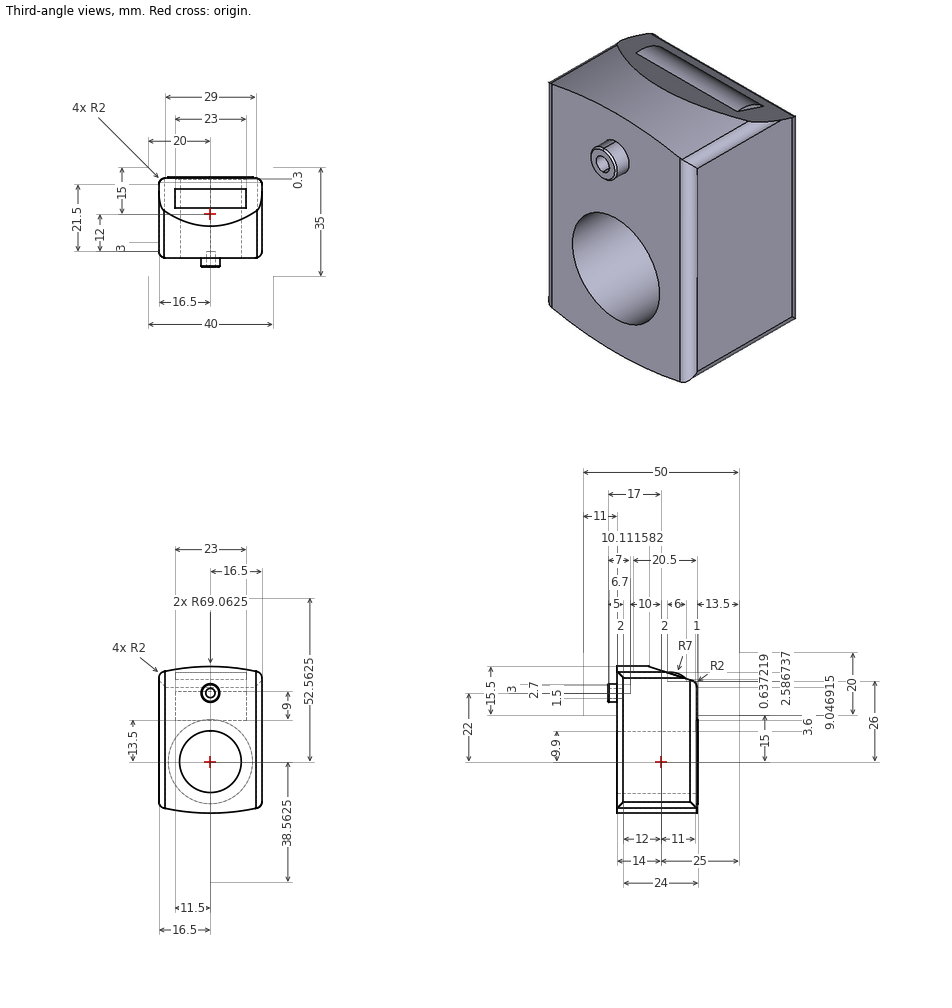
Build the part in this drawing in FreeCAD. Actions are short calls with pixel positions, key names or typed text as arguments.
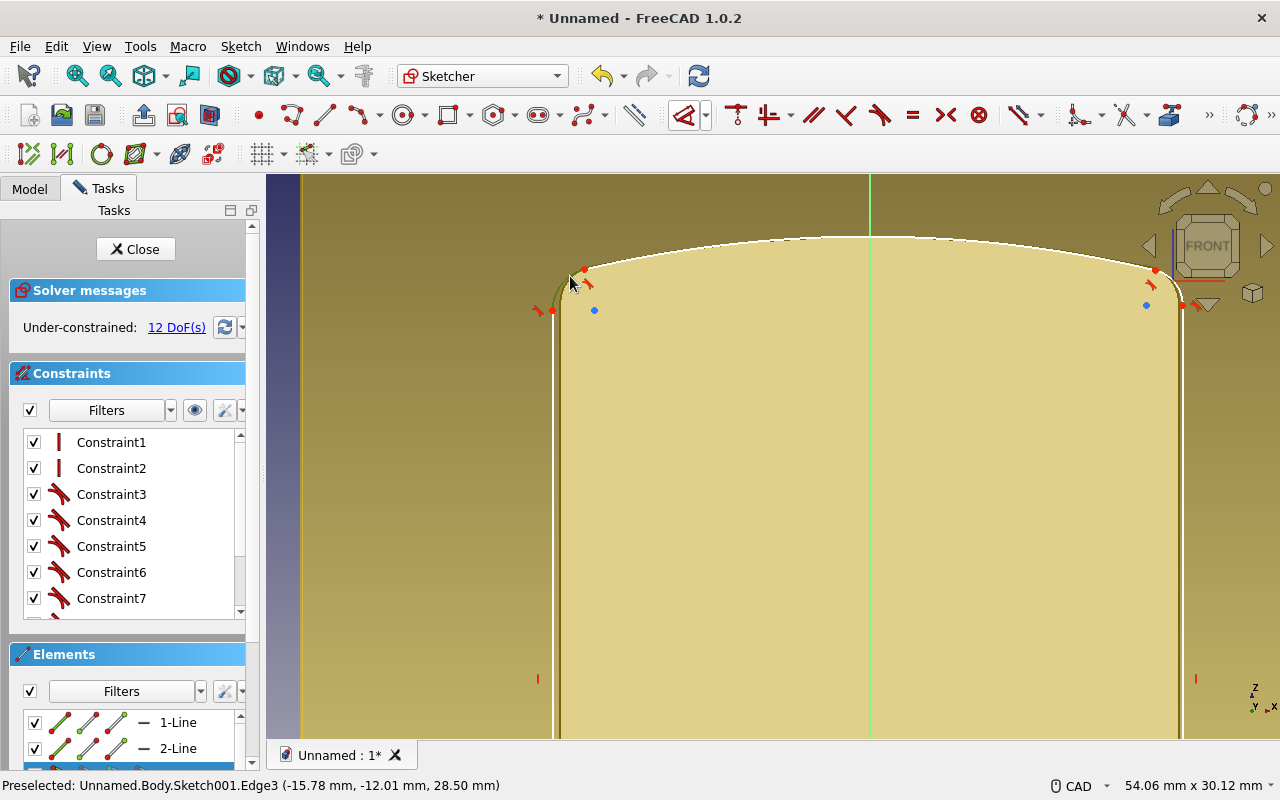
scroll(570, 276, down, 4)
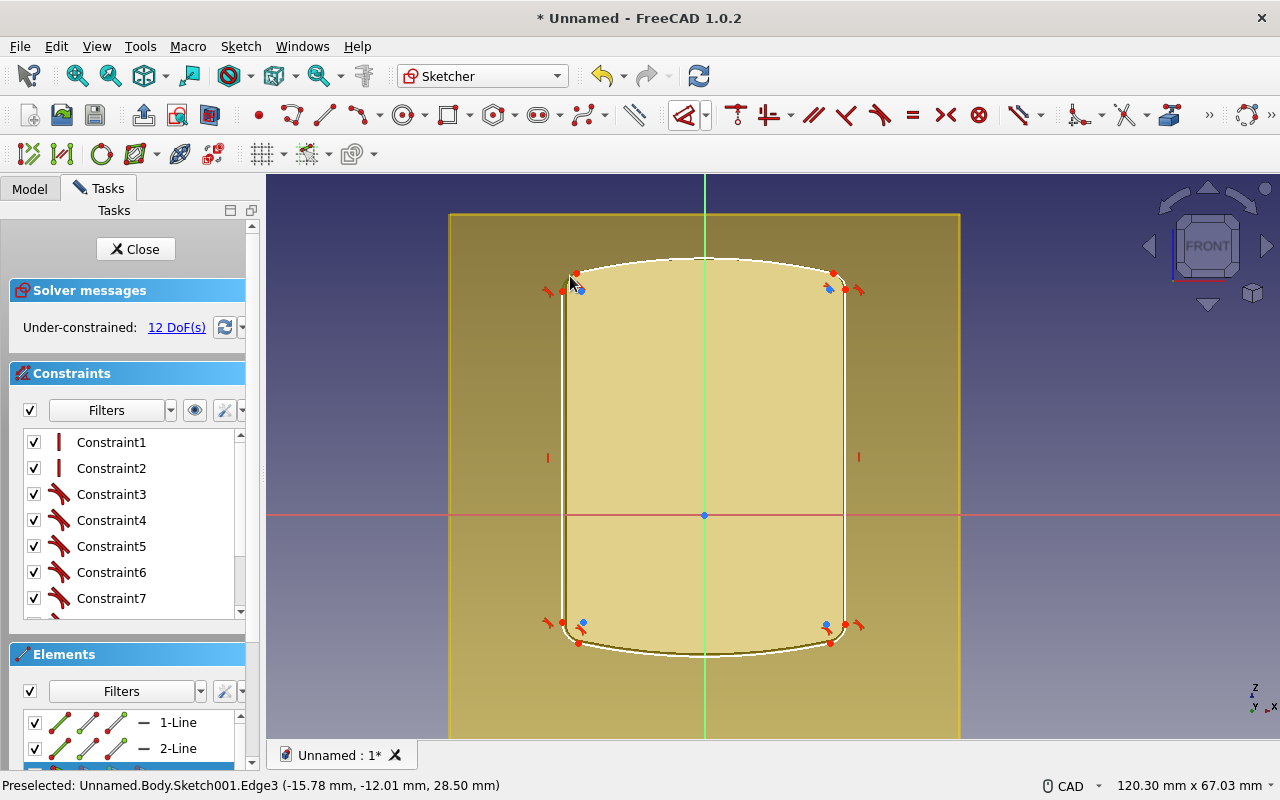
scroll(844, 283, up, 4)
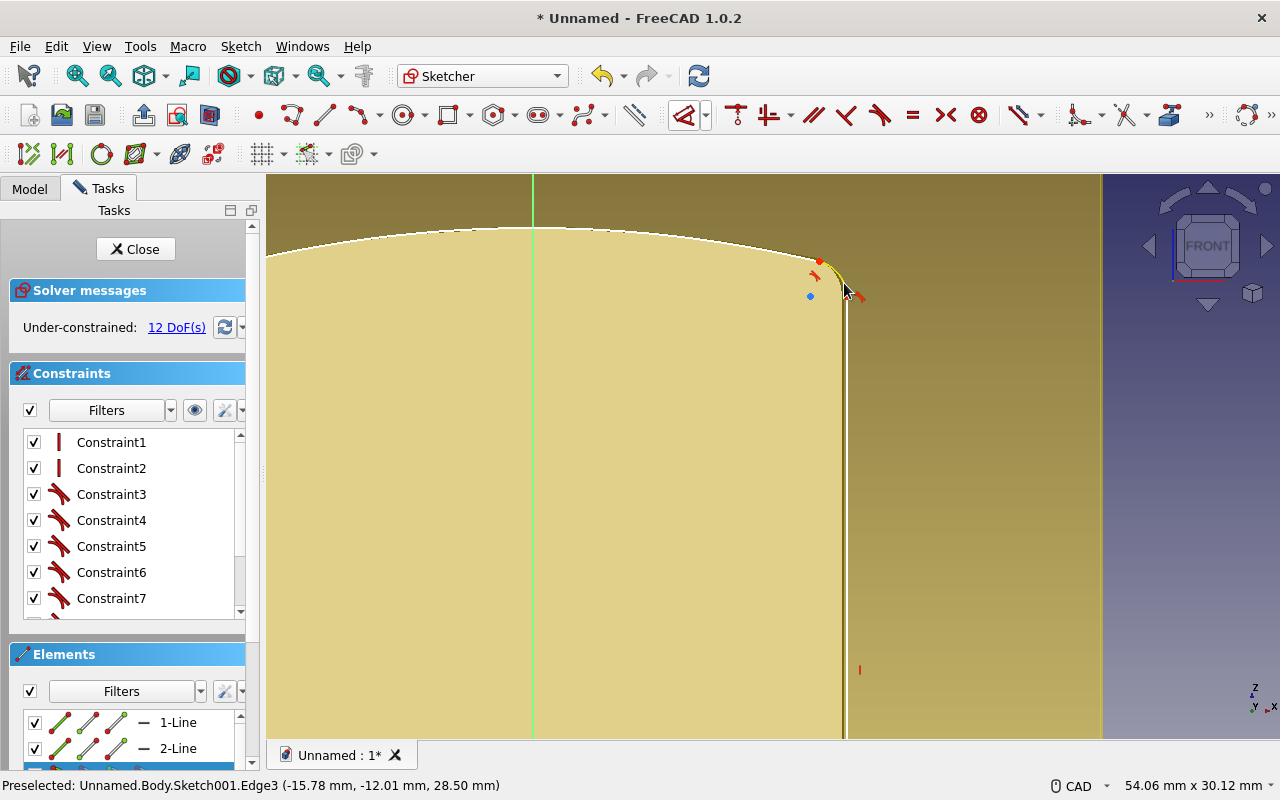
click(844, 283)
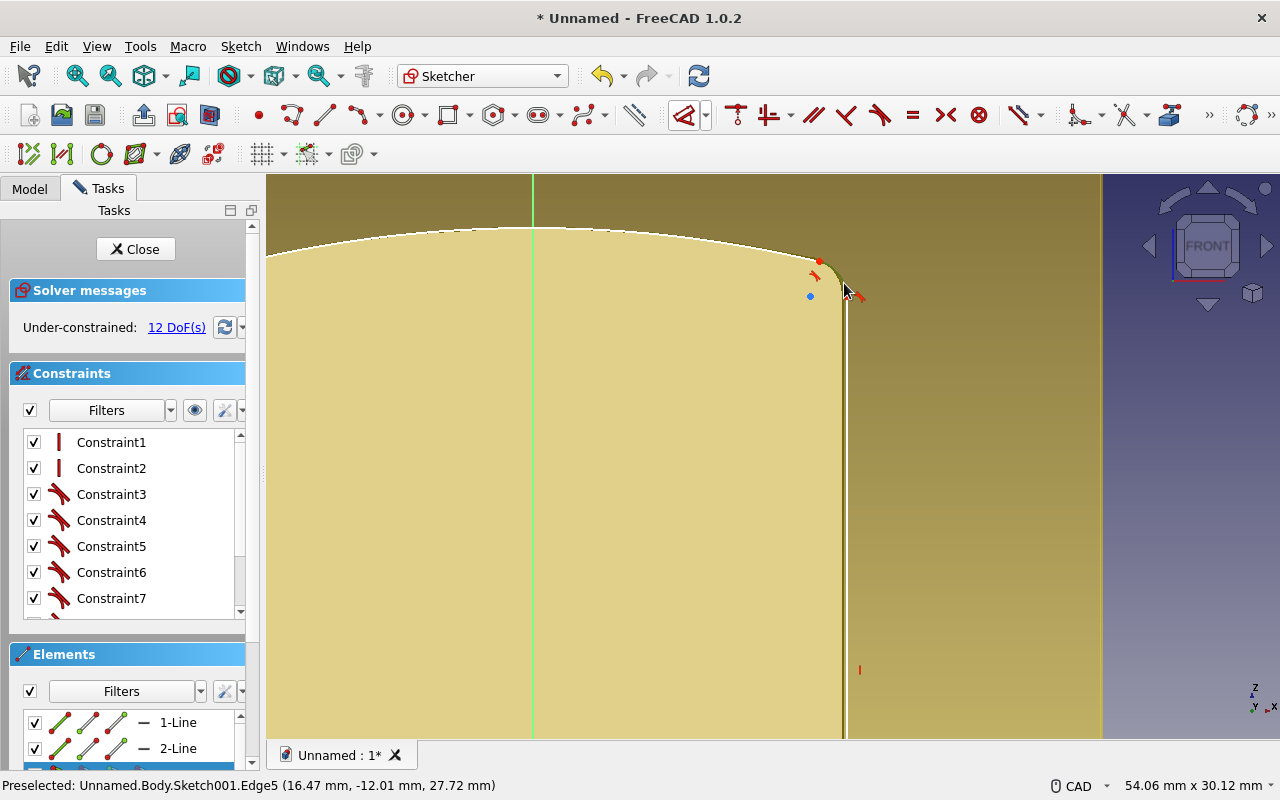
scroll(844, 283, down, 4)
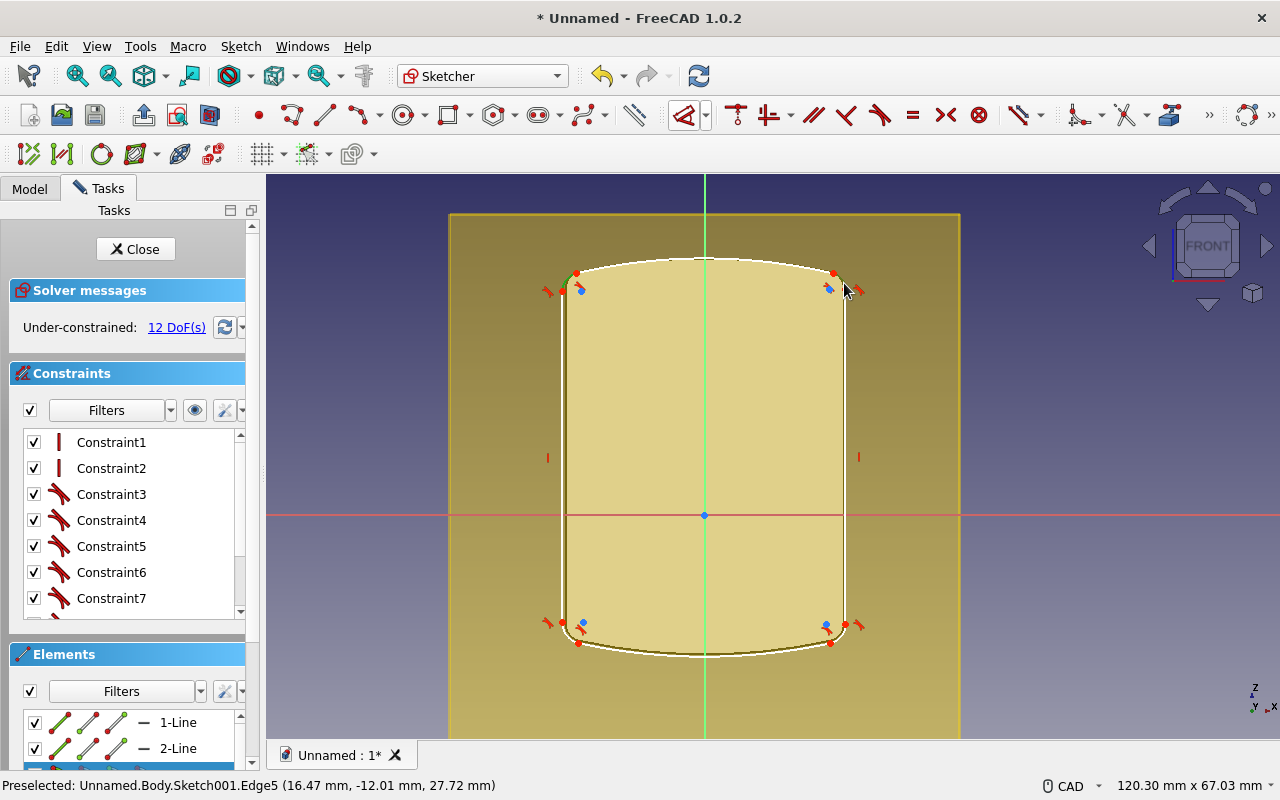
scroll(837, 640, up, 3)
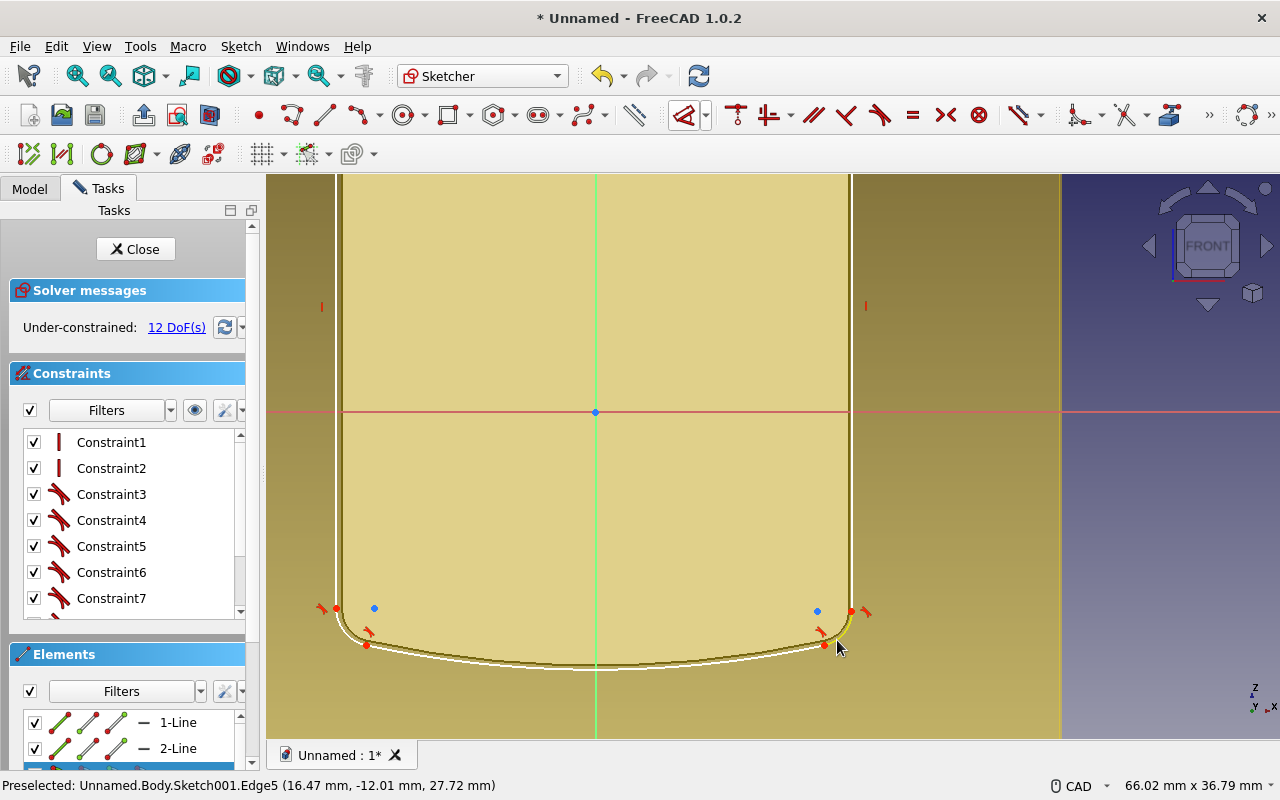
click(837, 640)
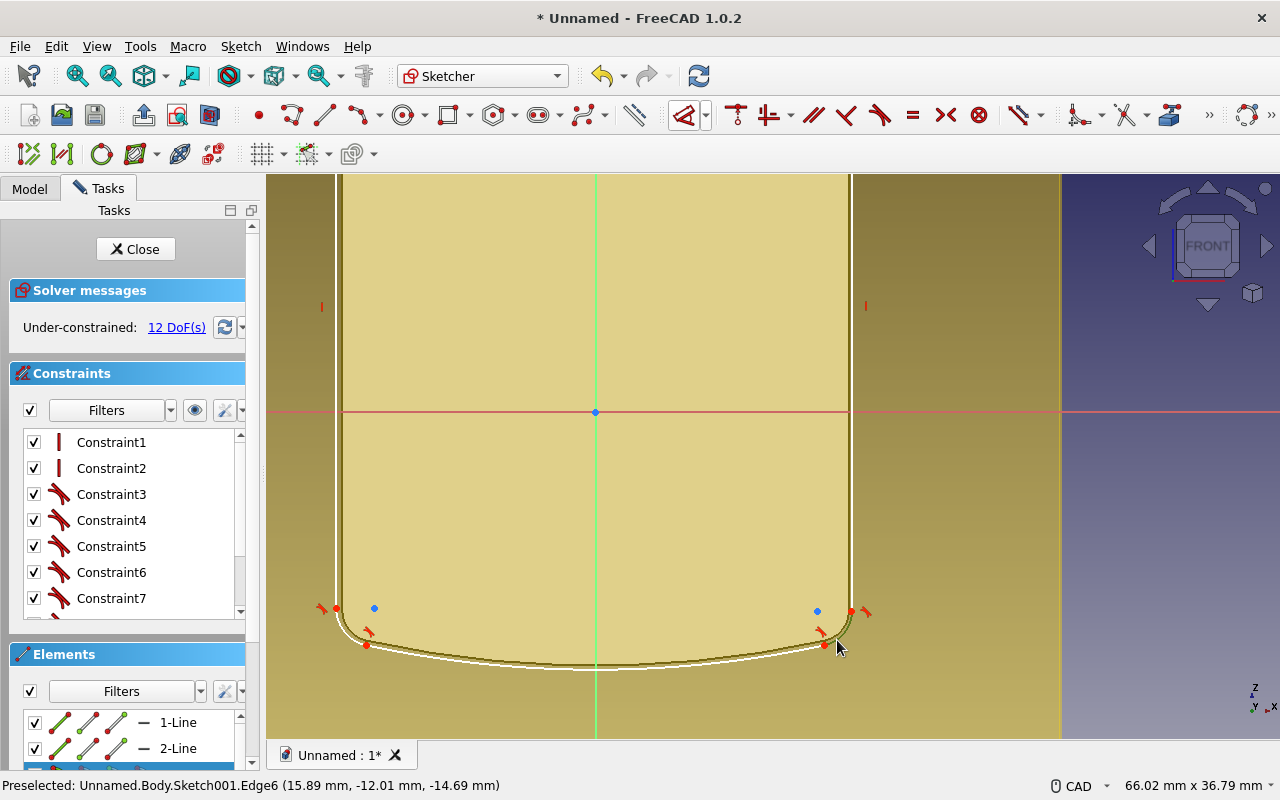
click(339, 623)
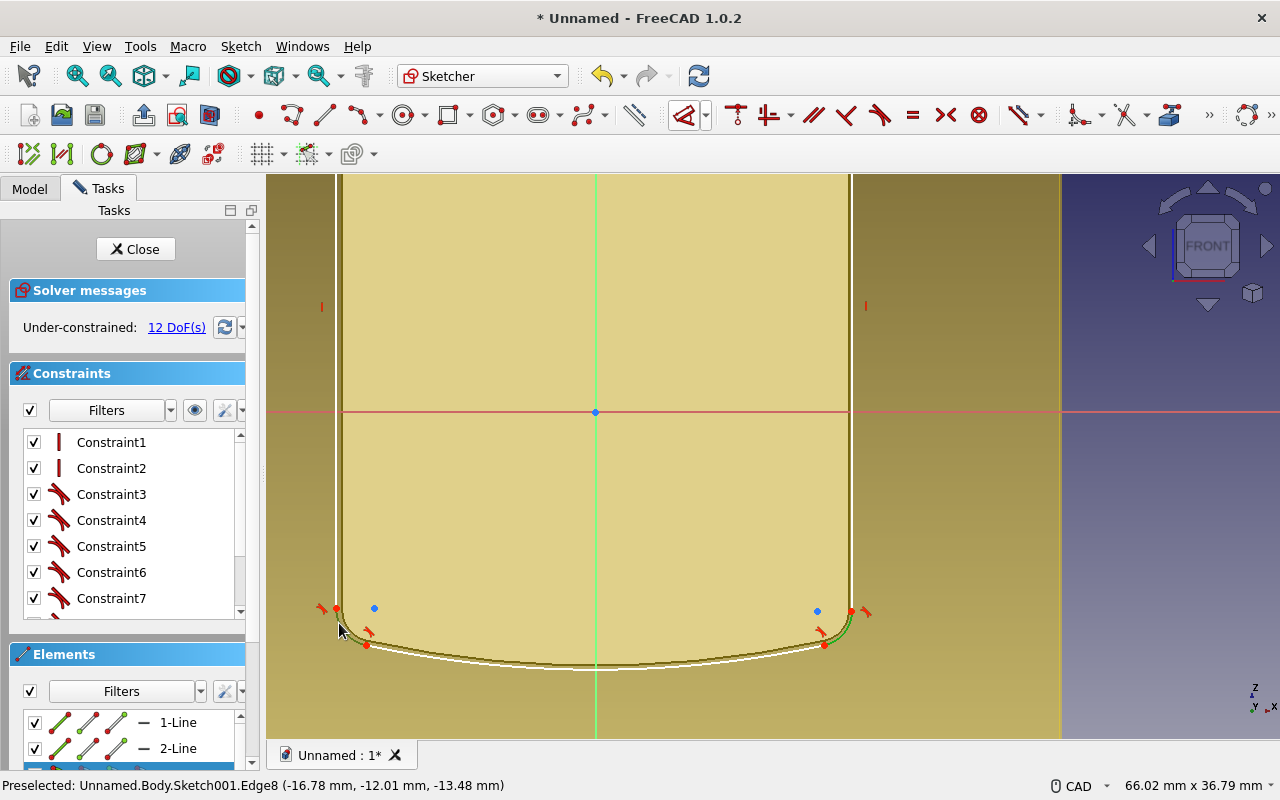
click(913, 116)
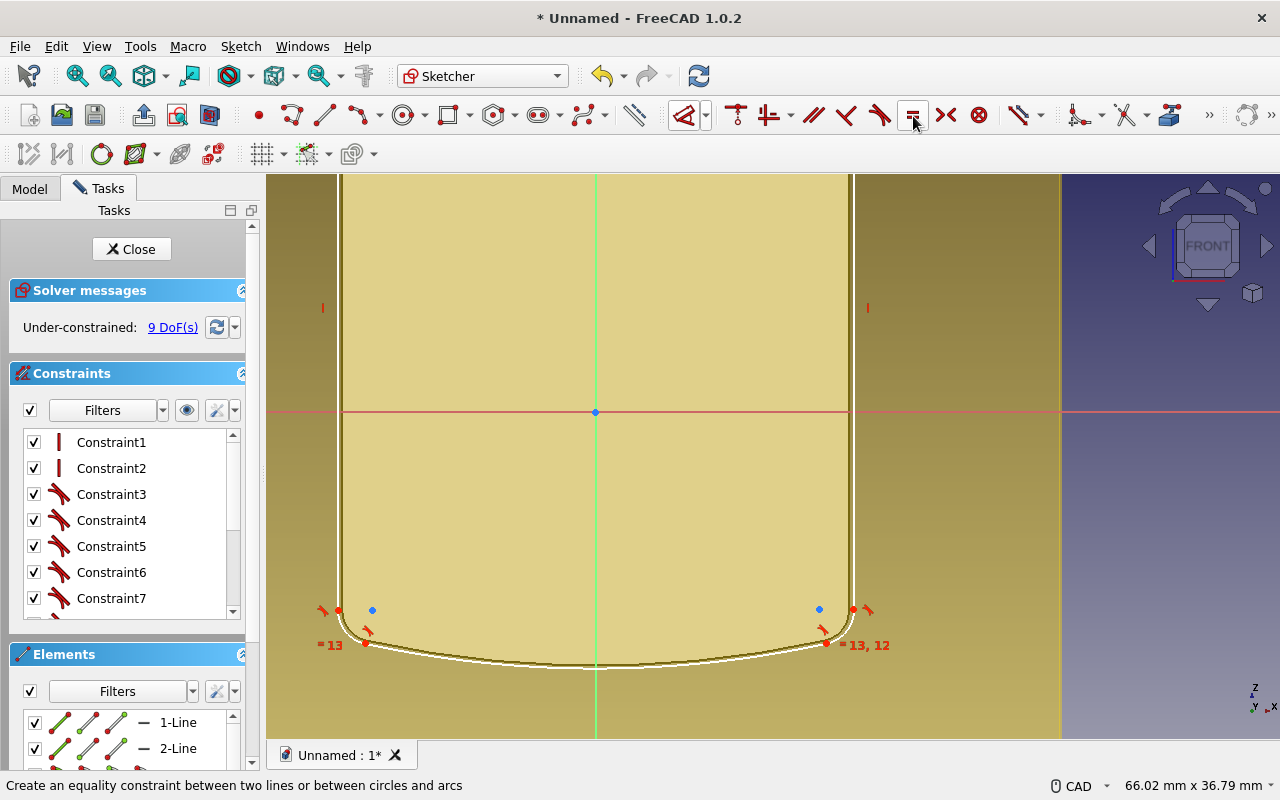
scroll(837, 641, down, 3)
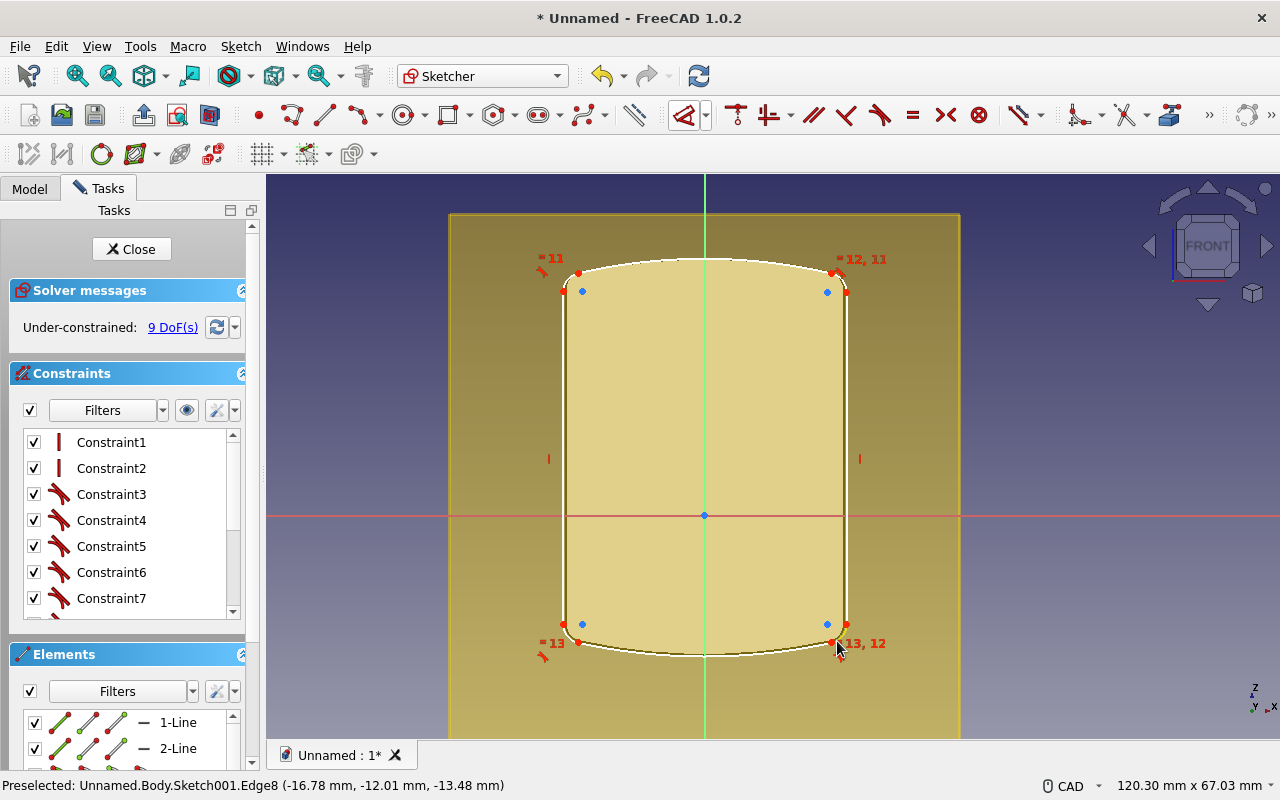
click(756, 261)